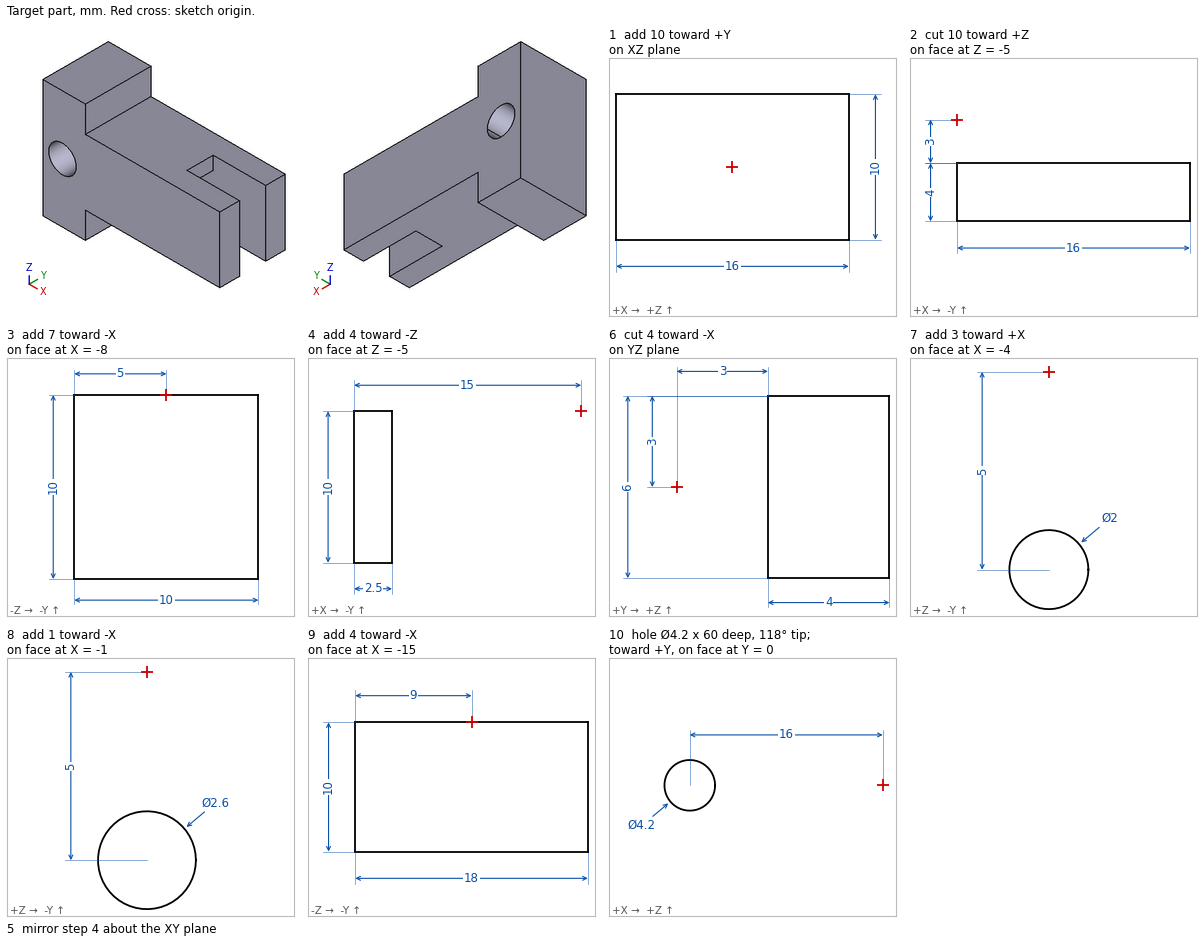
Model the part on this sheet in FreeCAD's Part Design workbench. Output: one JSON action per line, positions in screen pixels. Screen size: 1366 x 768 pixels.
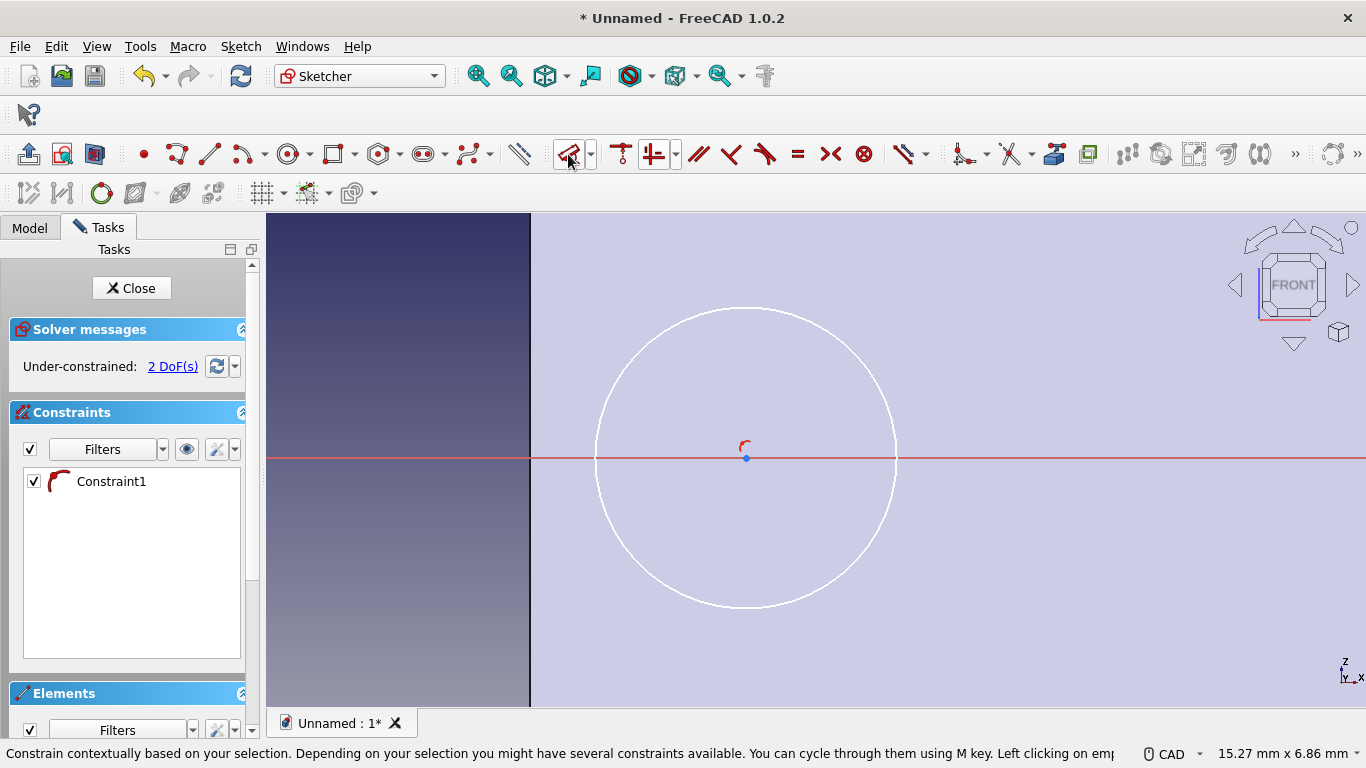
{"action": "left_click", "coordinate": [852, 351]}
{"action": "left_click", "coordinate": [875, 328]}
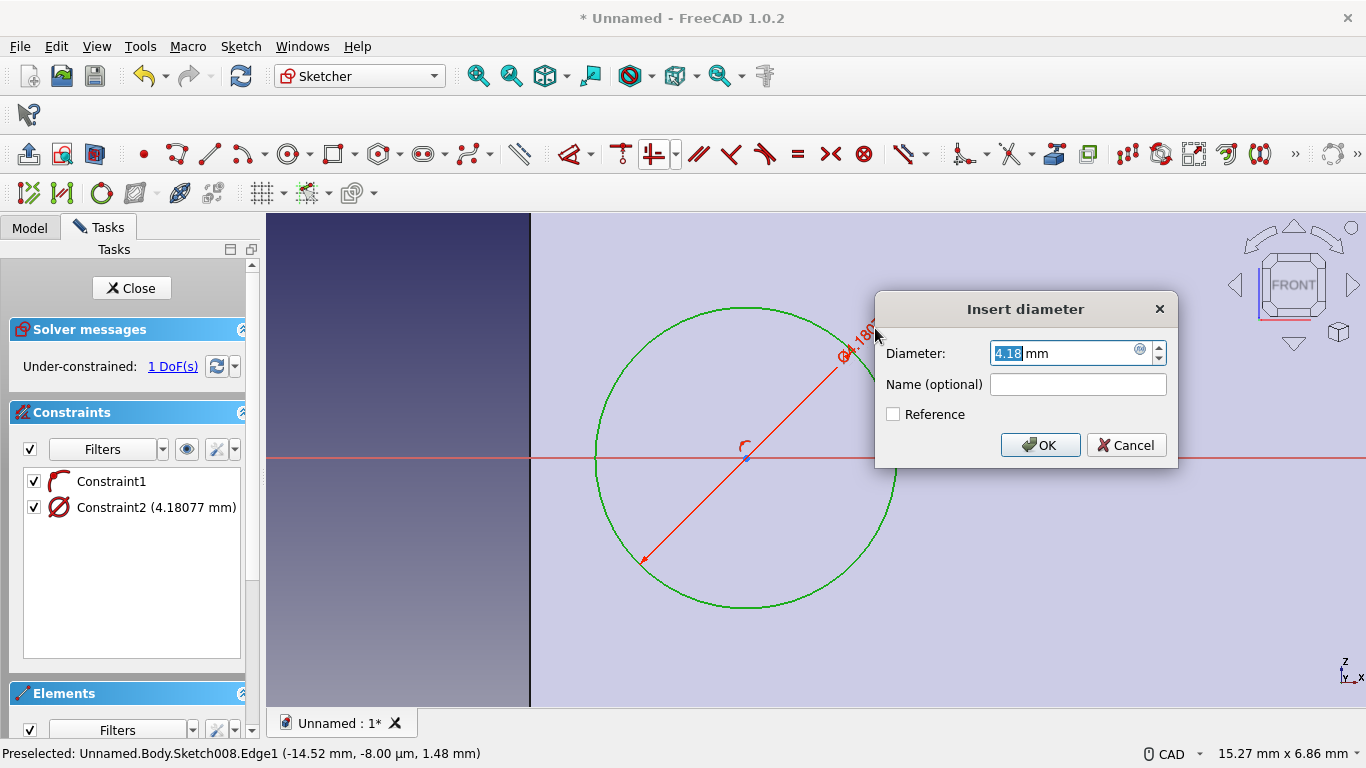
{"action": "type", "text": "4.2"}
{"action": "key", "text": "Return"}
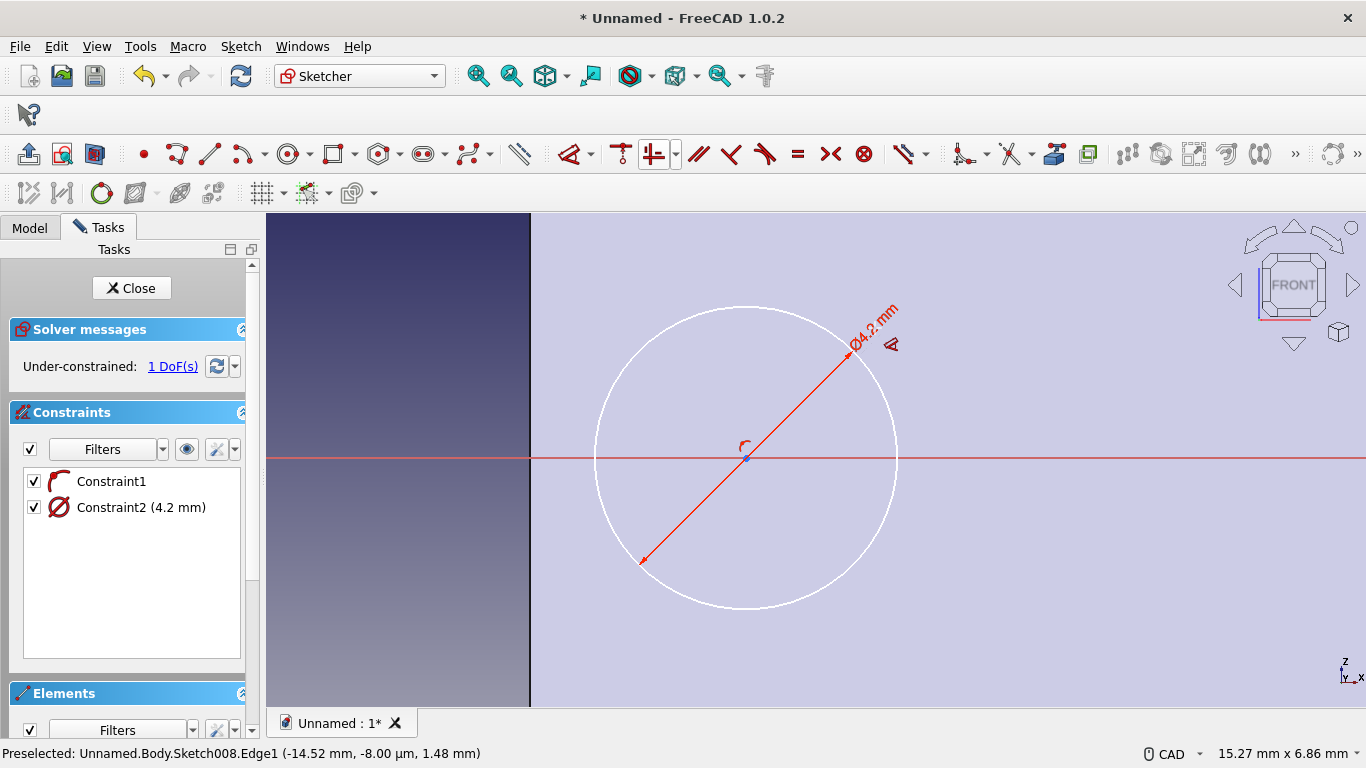
{"action": "left_click", "coordinate": [746, 458]}
{"action": "left_click", "coordinate": [973, 492]}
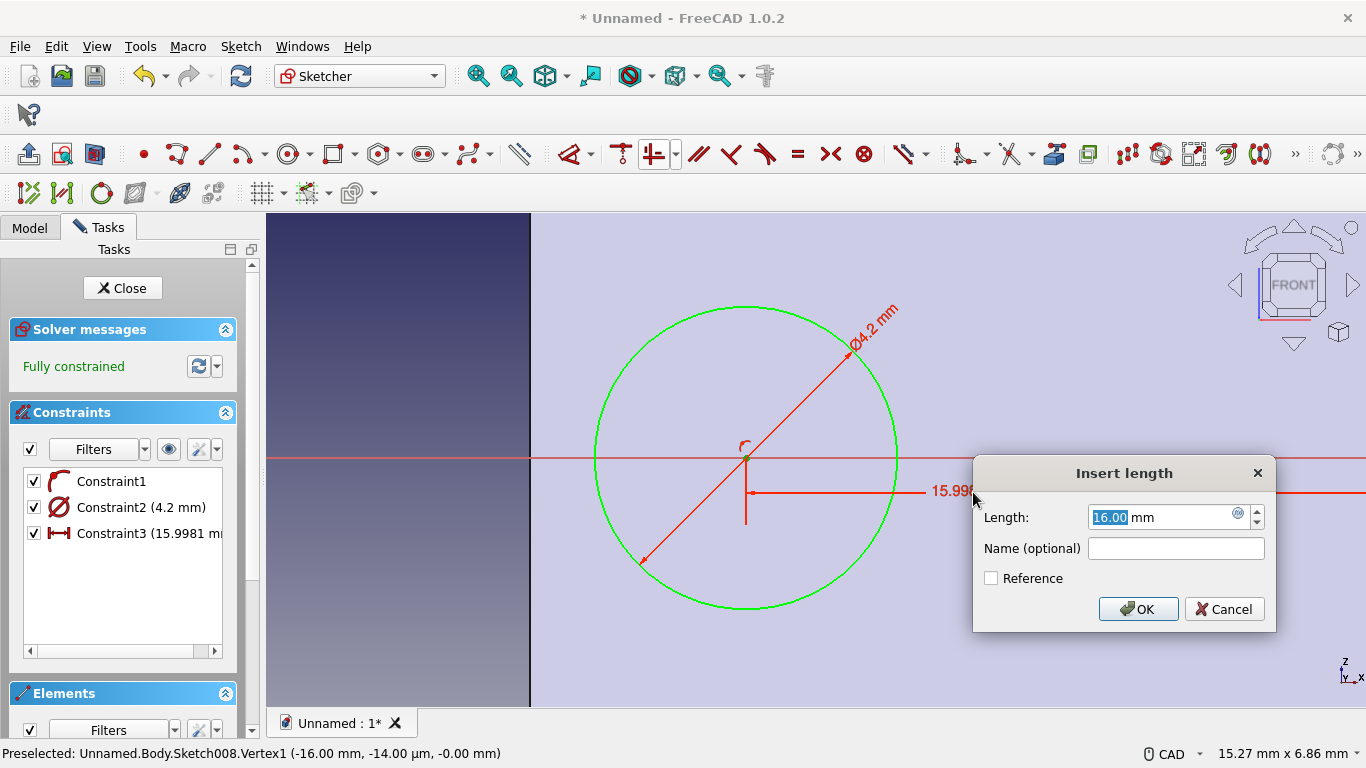
{"action": "type", "text": "16"}
{"action": "key", "text": "Return"}
{"action": "key", "text": "Escape"}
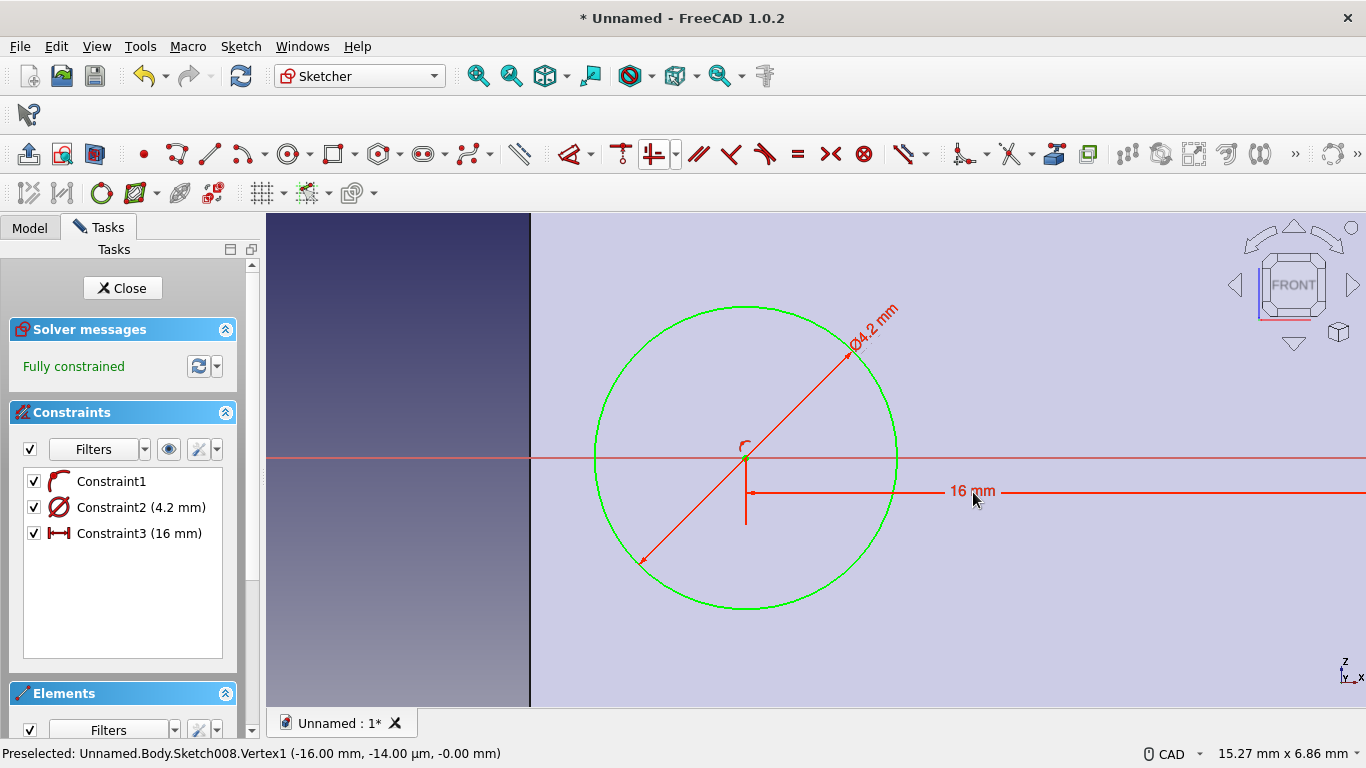
{"action": "left_click", "coordinate": [123, 288]}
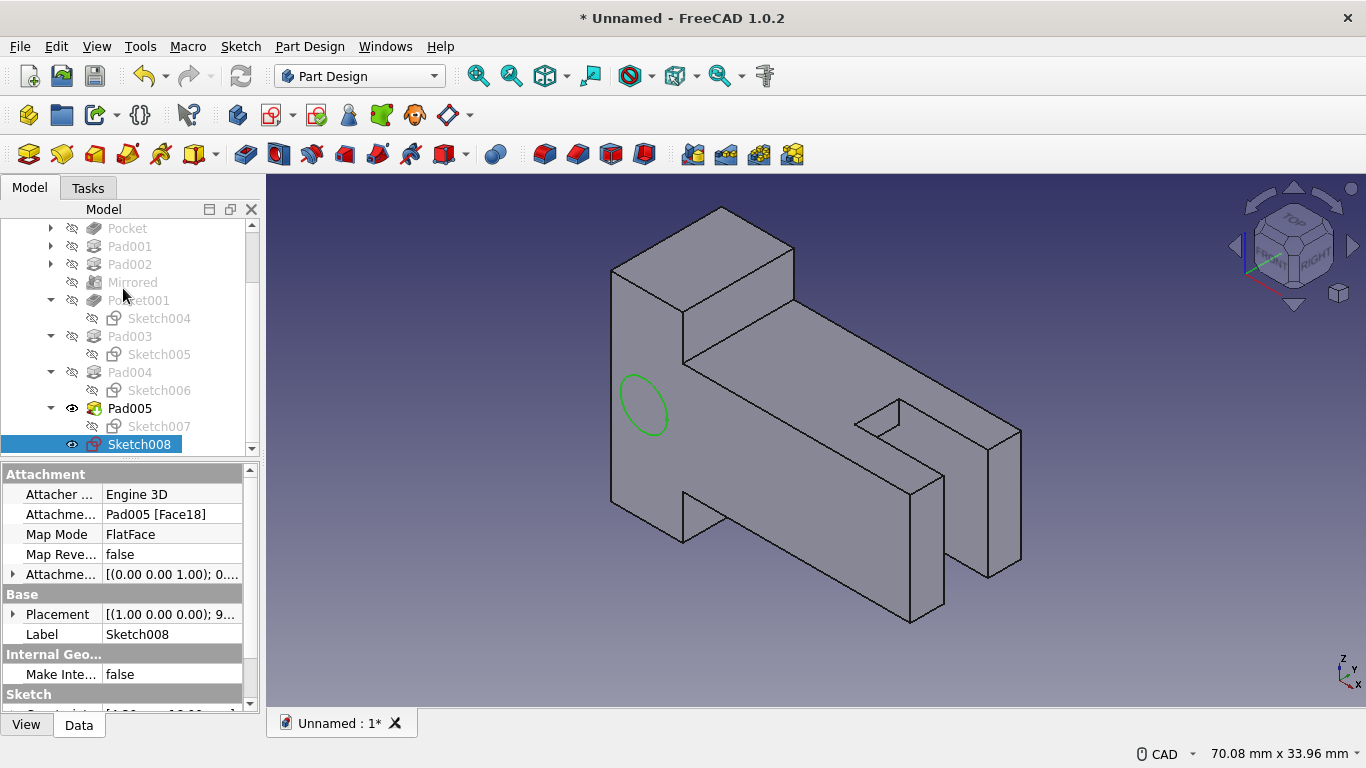
{"action": "left_click", "coordinate": [279, 154]}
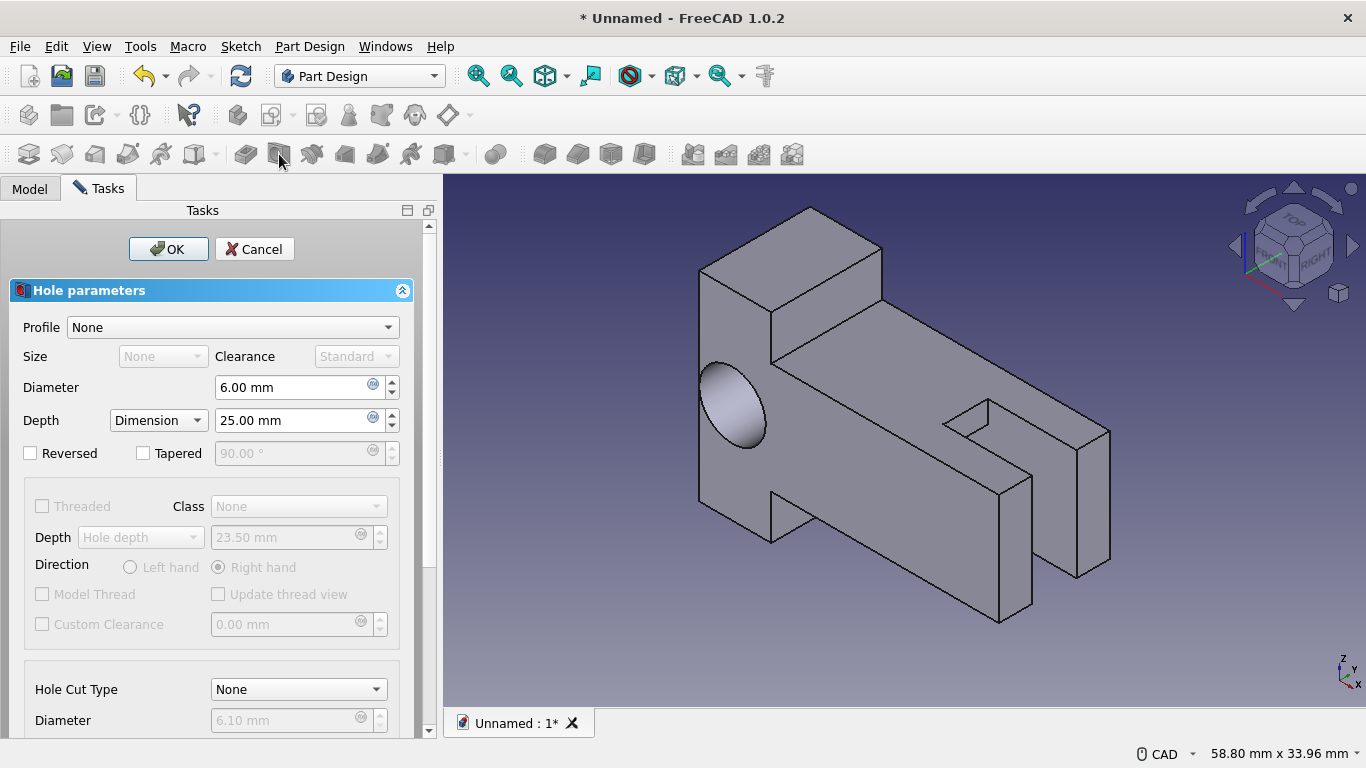
{"action": "triple_click", "coordinate": [300, 388]}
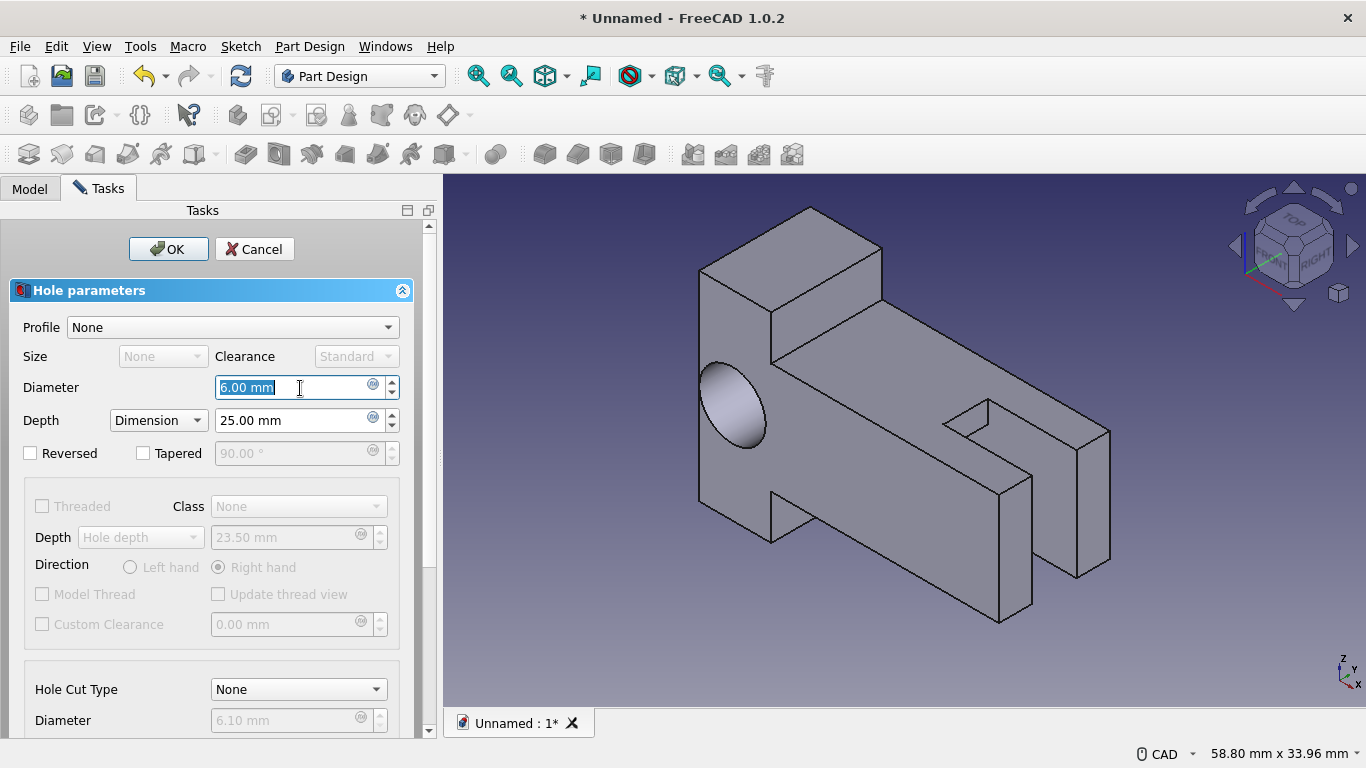
{"action": "type", "text": "4.2"}
{"action": "key", "text": "Tab"}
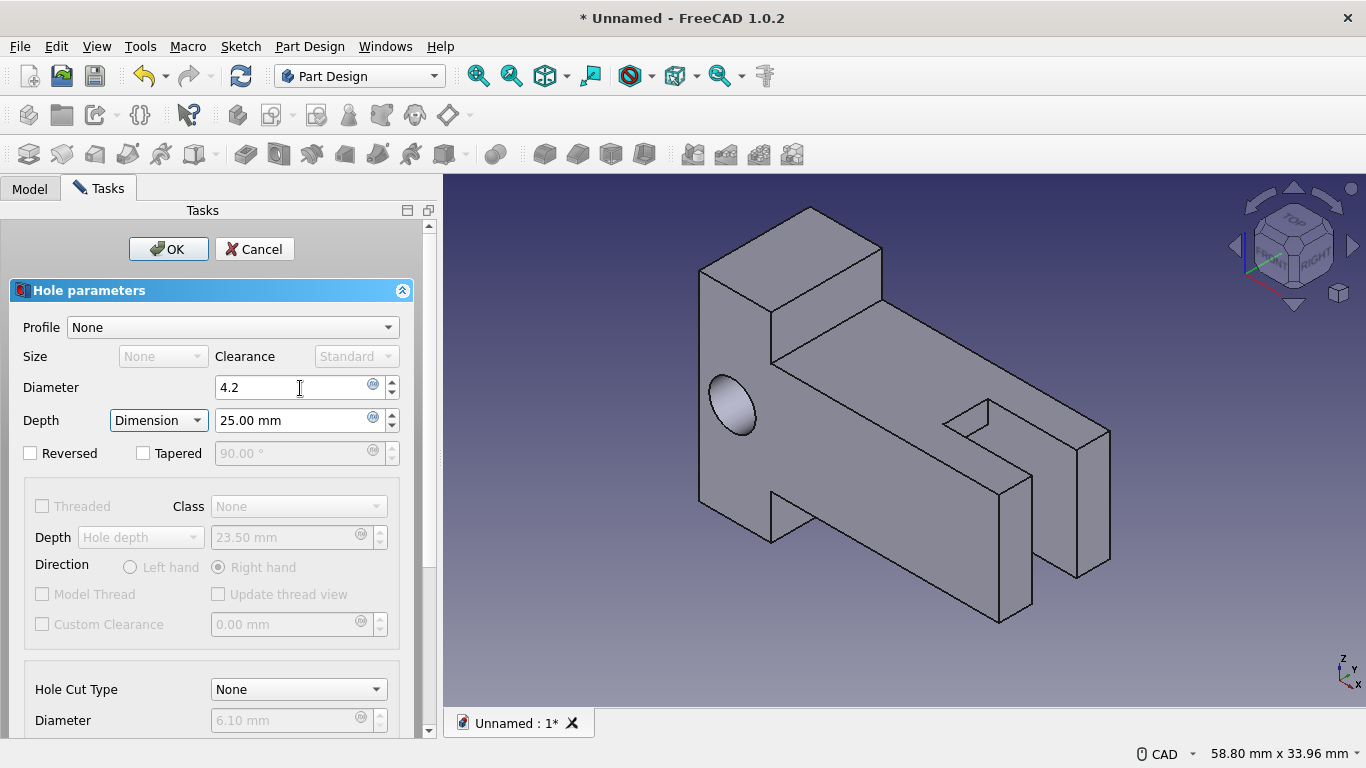
{"action": "triple_click", "coordinate": [300, 420]}